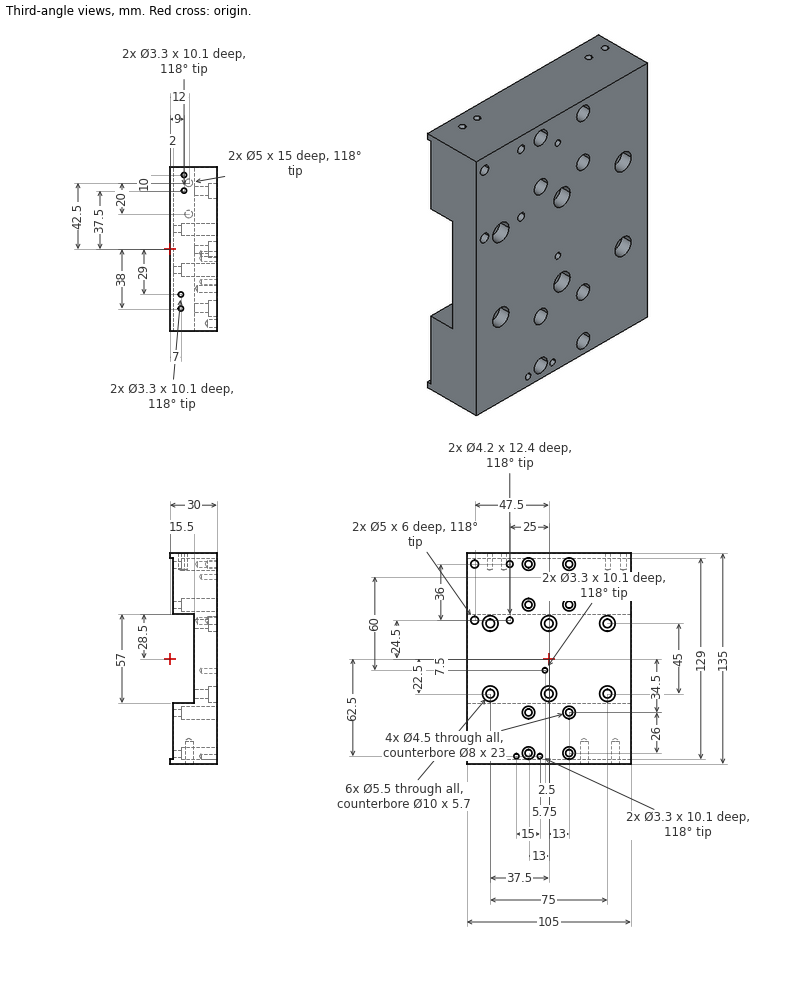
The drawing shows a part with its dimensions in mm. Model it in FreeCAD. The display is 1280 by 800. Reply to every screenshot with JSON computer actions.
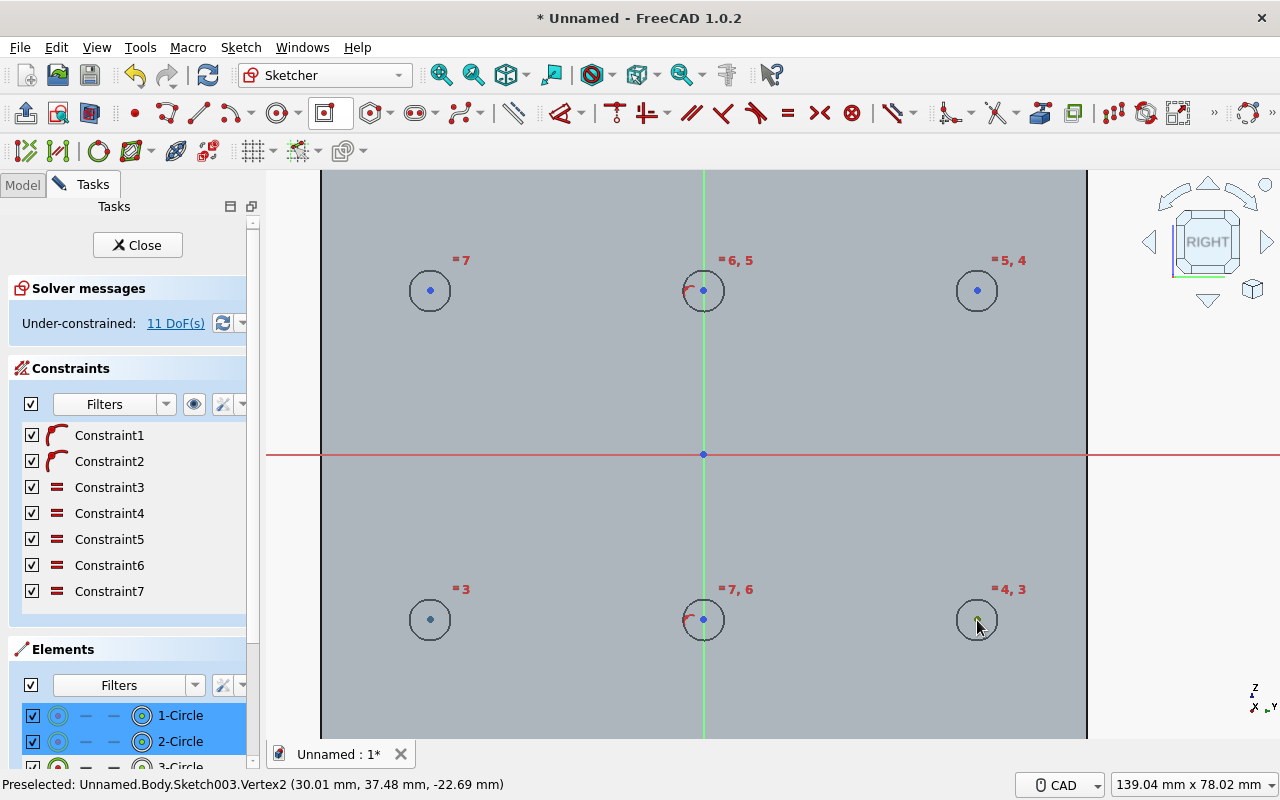
{"action": "left_click", "coordinate": [670, 114]}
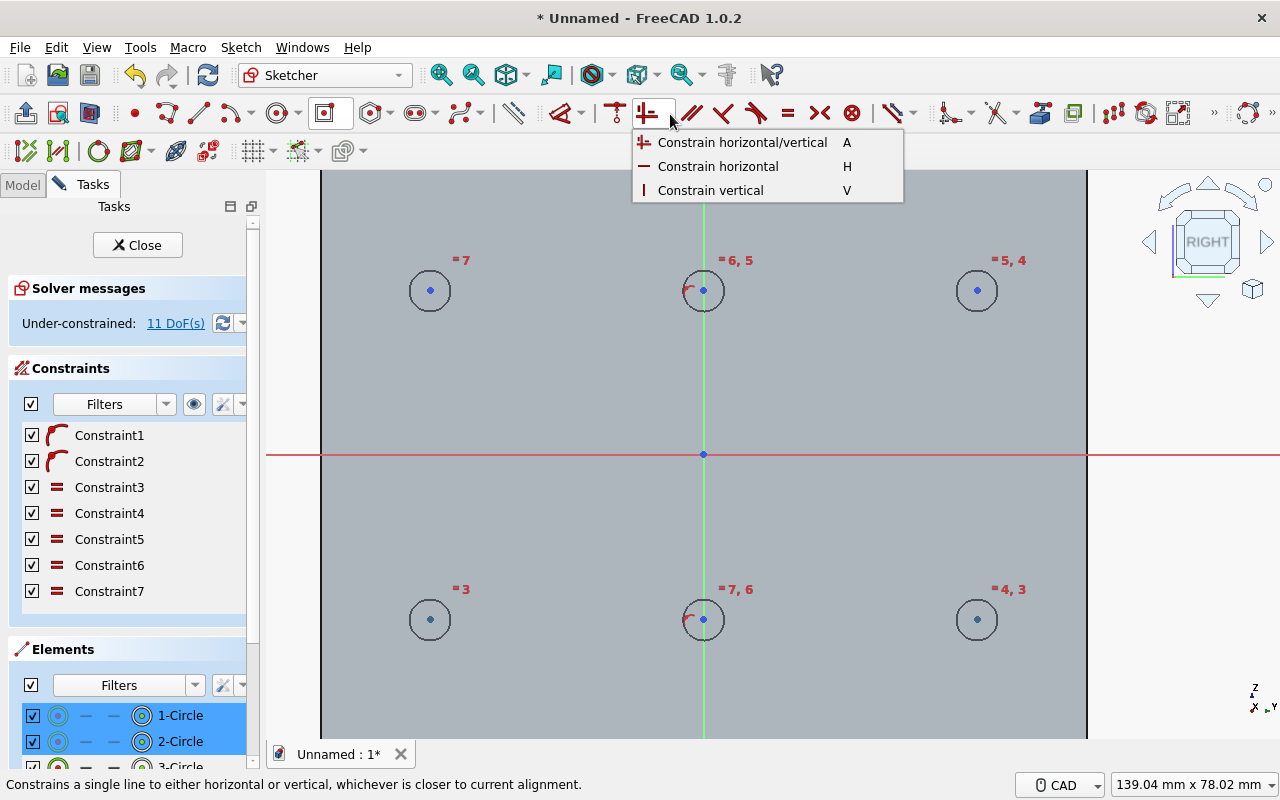
{"action": "left_click", "coordinate": [768, 166]}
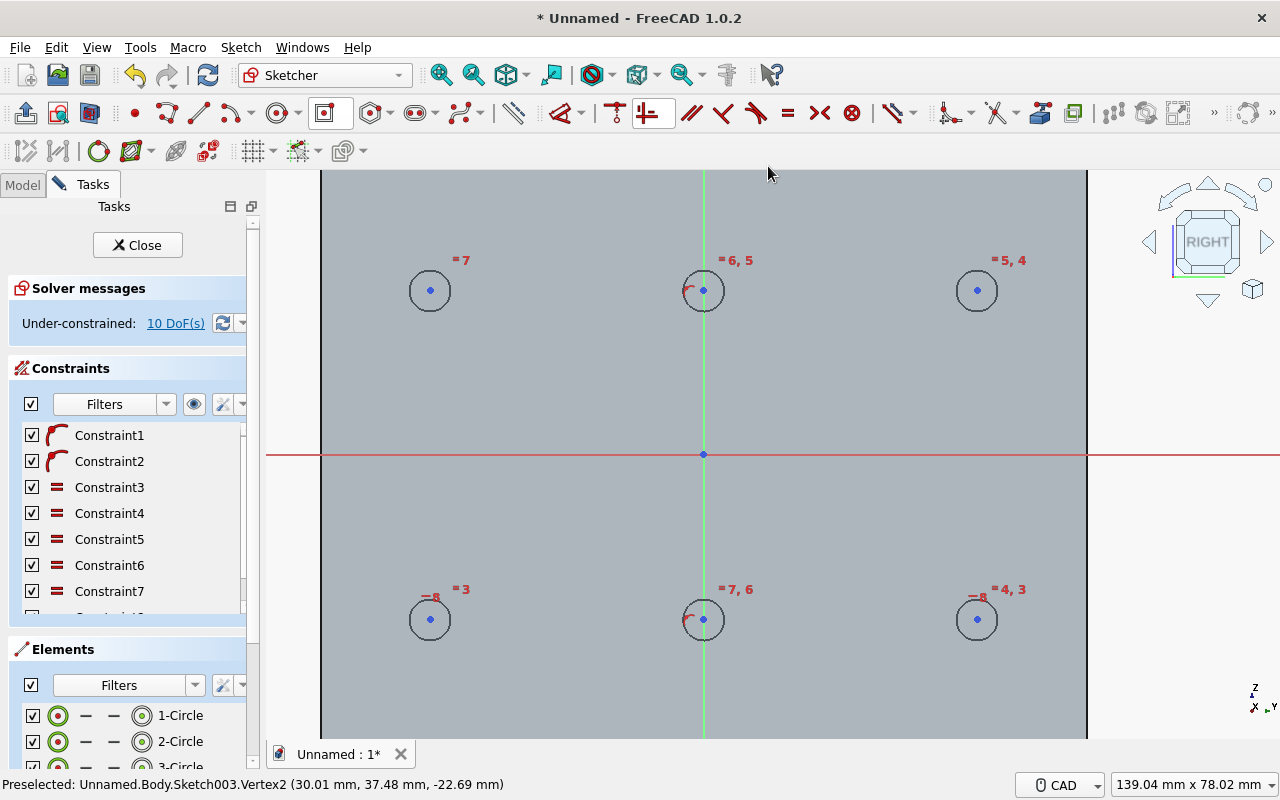
{"action": "left_click", "coordinate": [977, 620]}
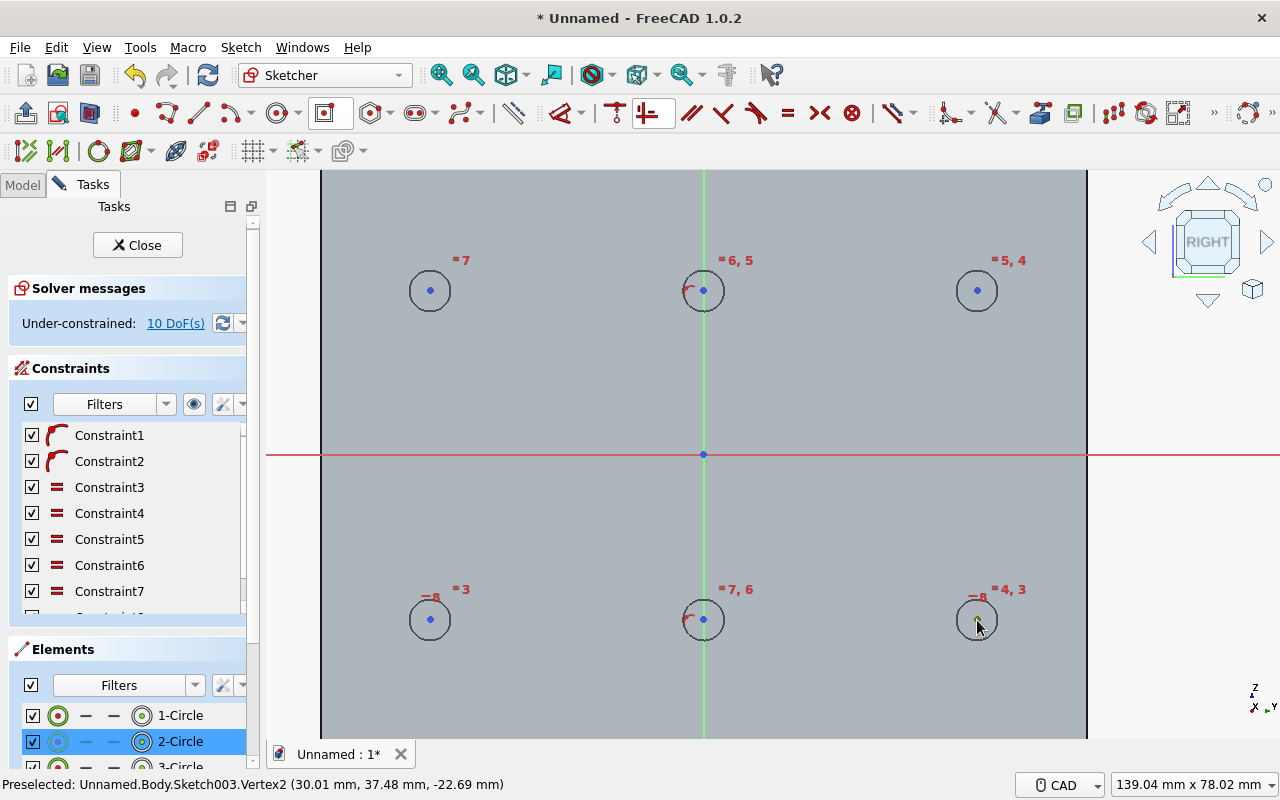
{"action": "left_click", "coordinate": [977, 291]}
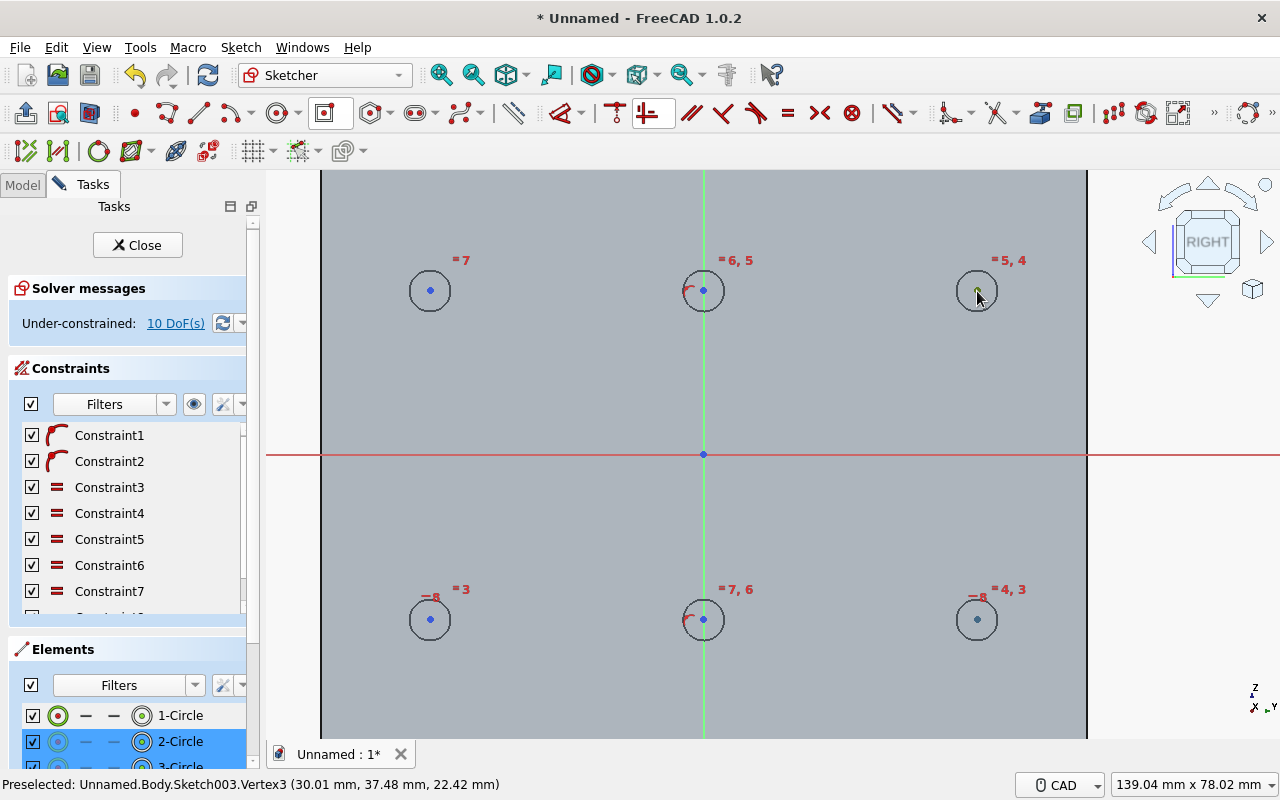
{"action": "key", "text": "v"}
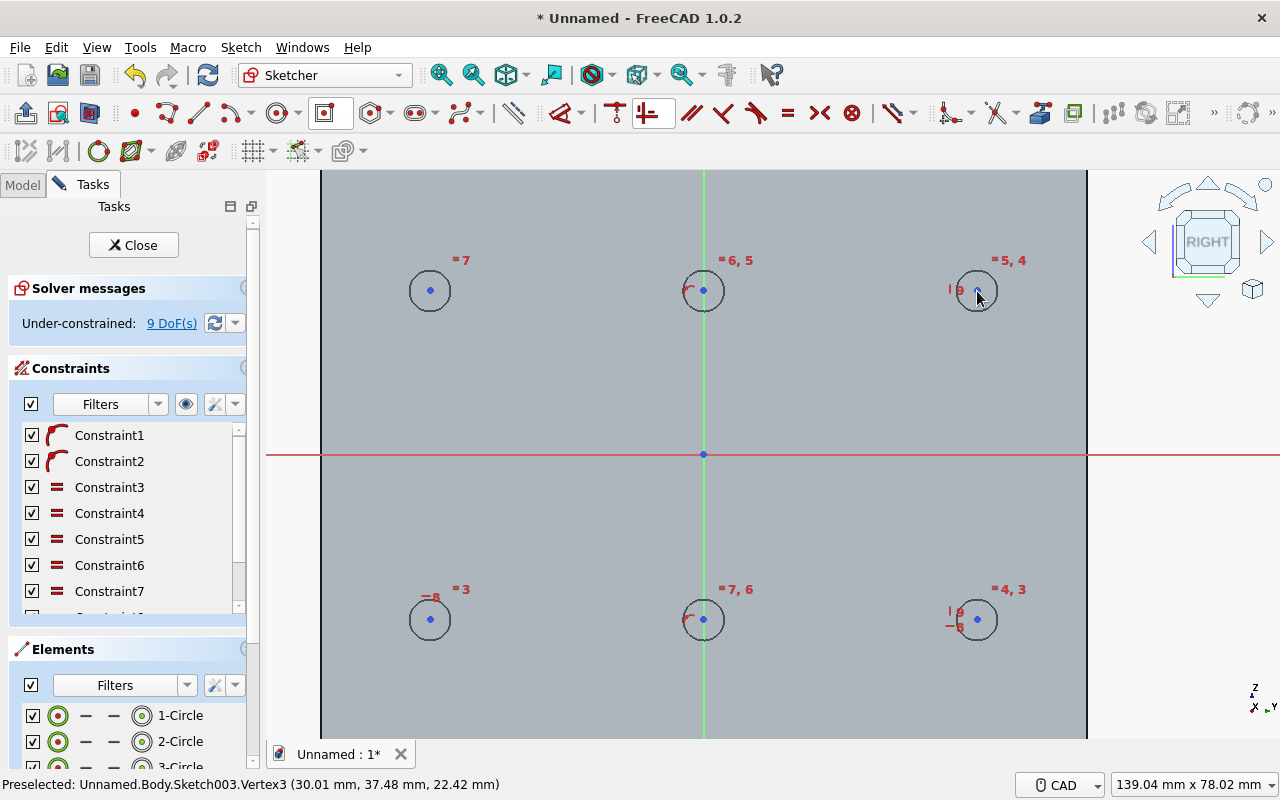
{"action": "left_click", "coordinate": [977, 291]}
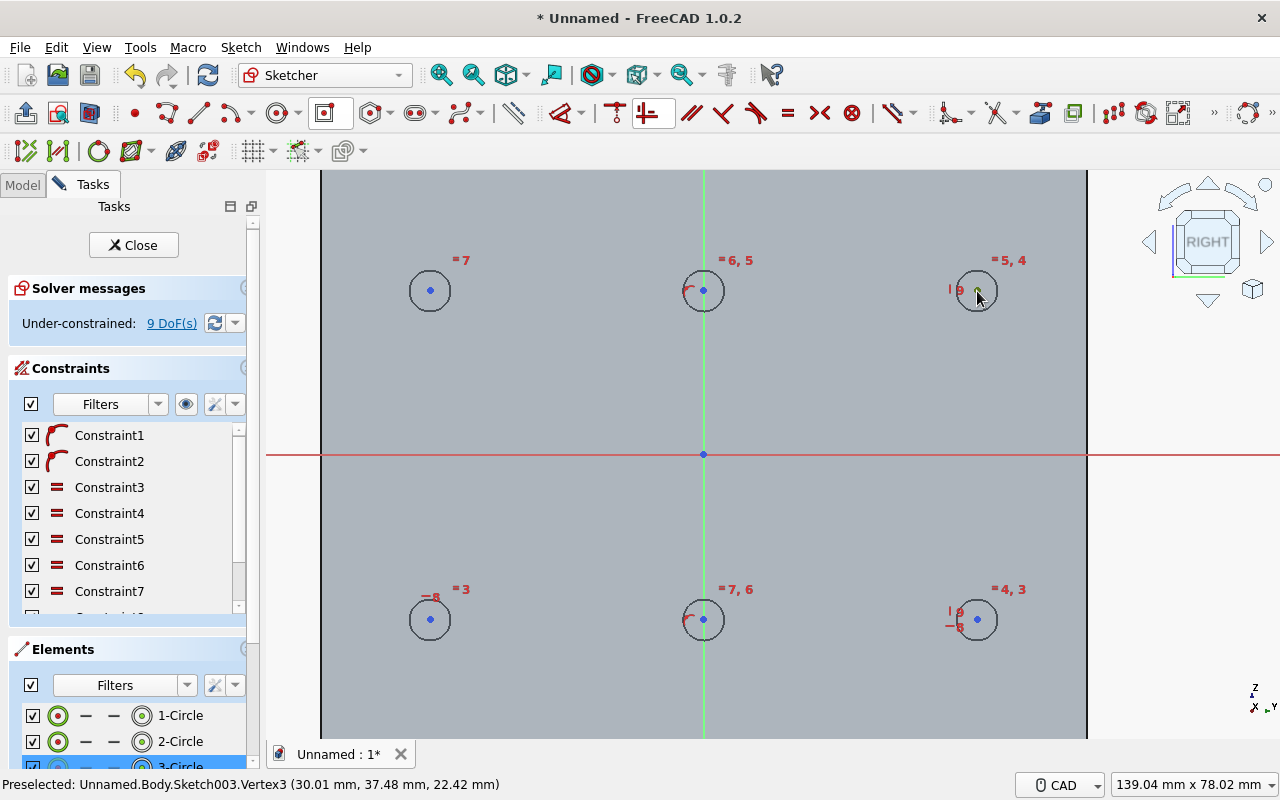
{"action": "left_click", "coordinate": [704, 291]}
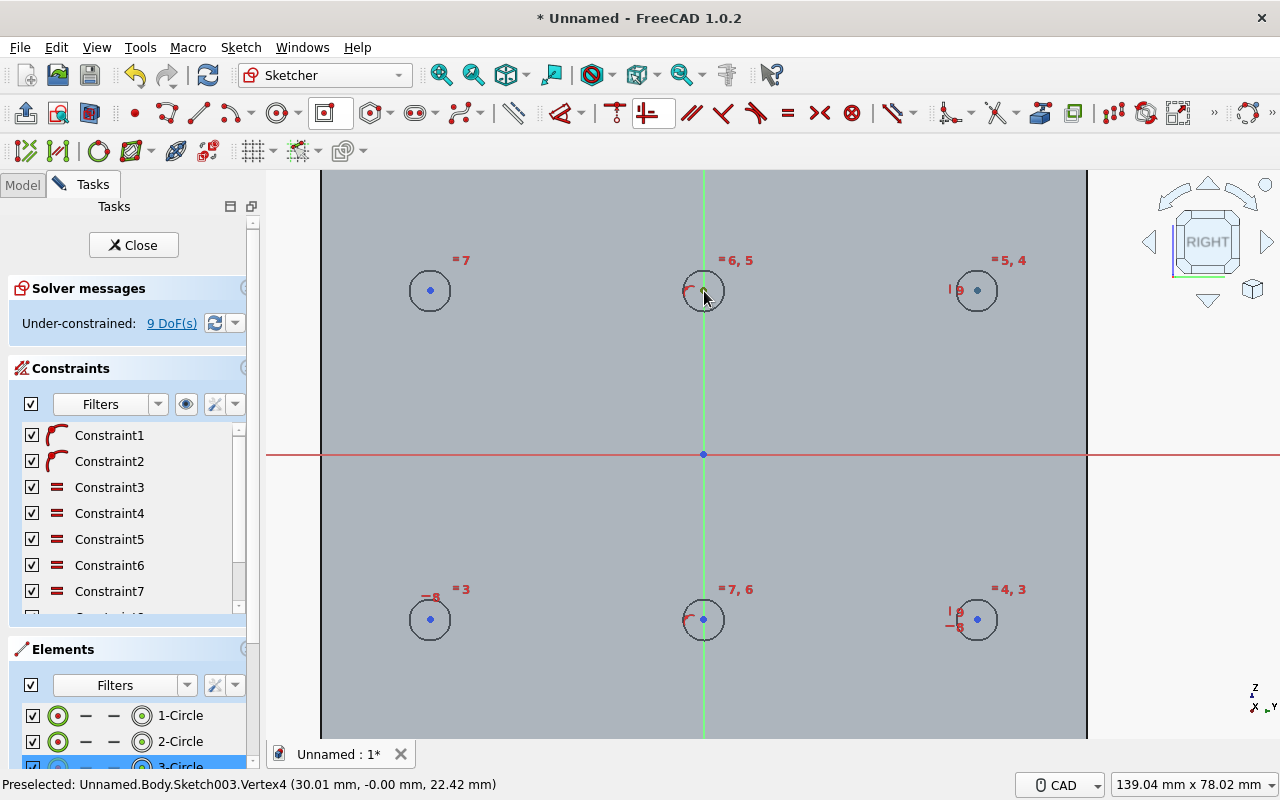
{"action": "left_click", "coordinate": [670, 114]}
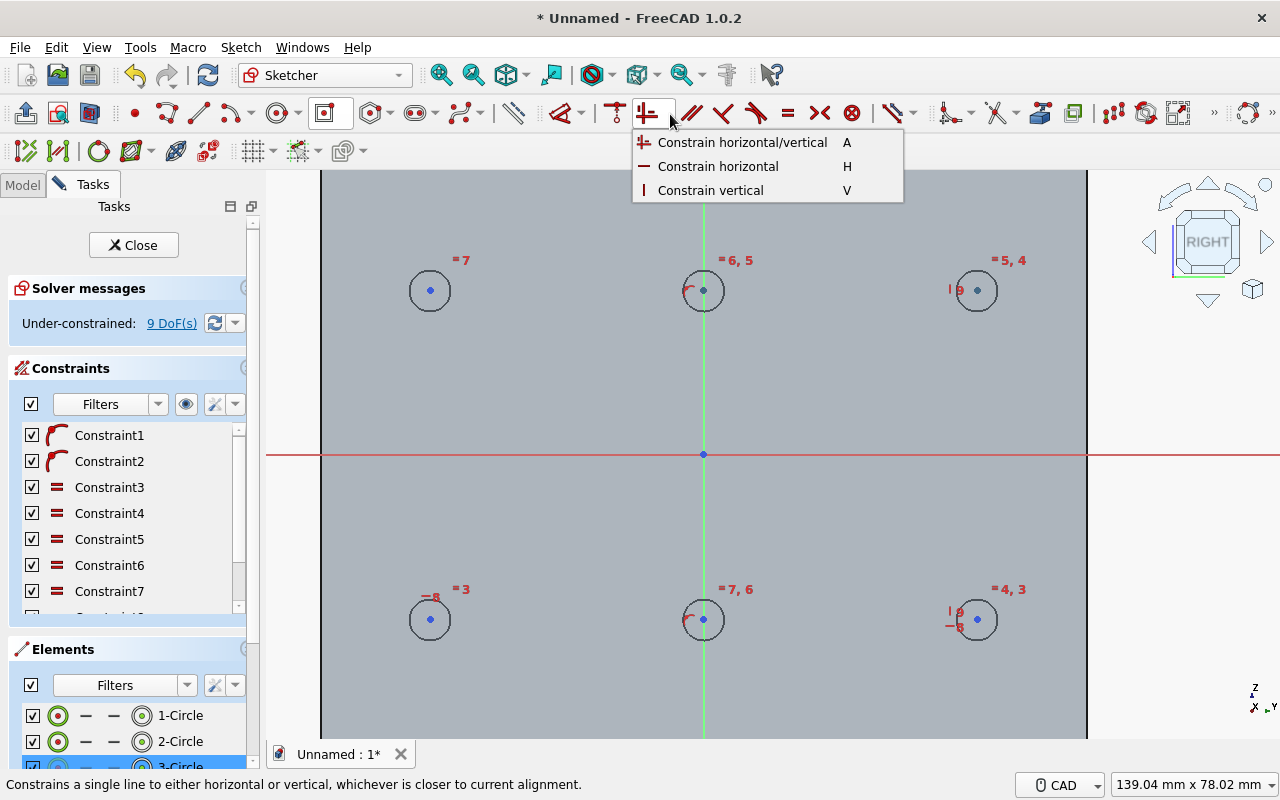
{"action": "left_click", "coordinate": [768, 166]}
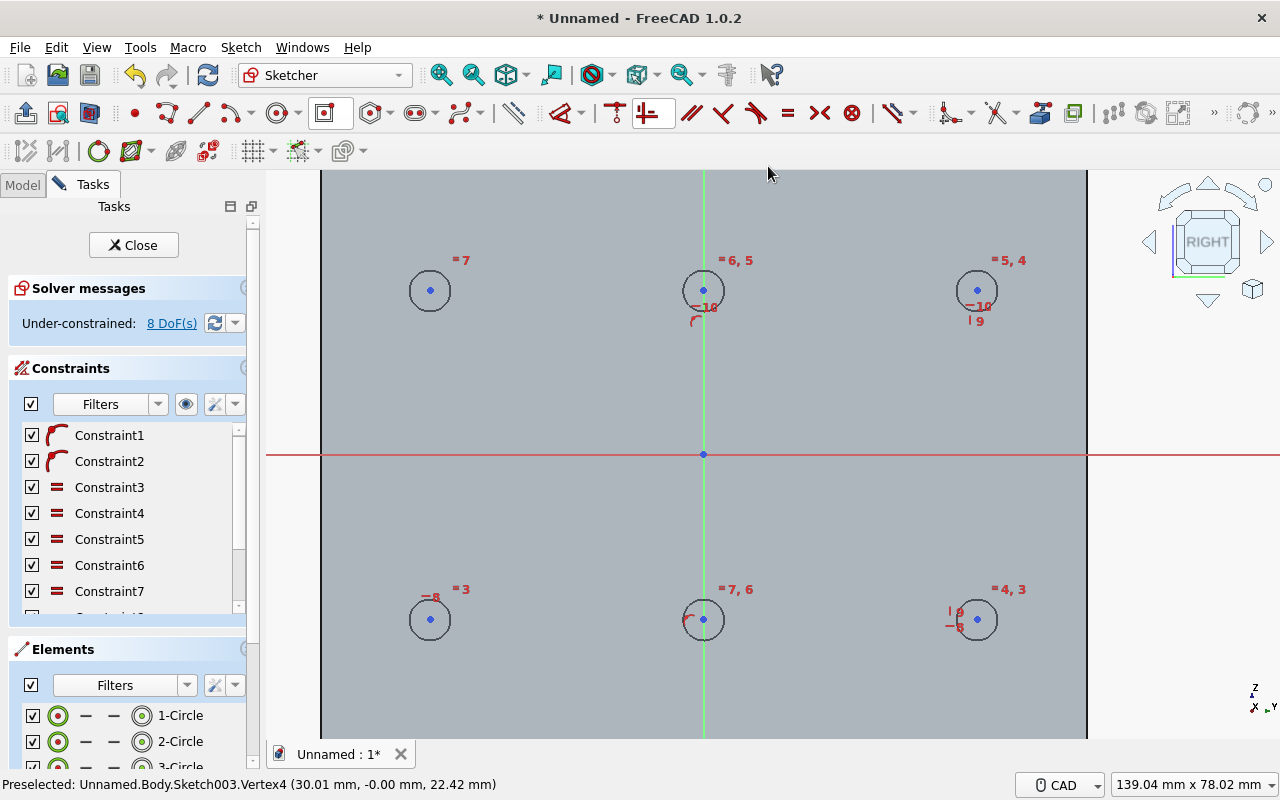
{"action": "left_click", "coordinate": [430, 620]}